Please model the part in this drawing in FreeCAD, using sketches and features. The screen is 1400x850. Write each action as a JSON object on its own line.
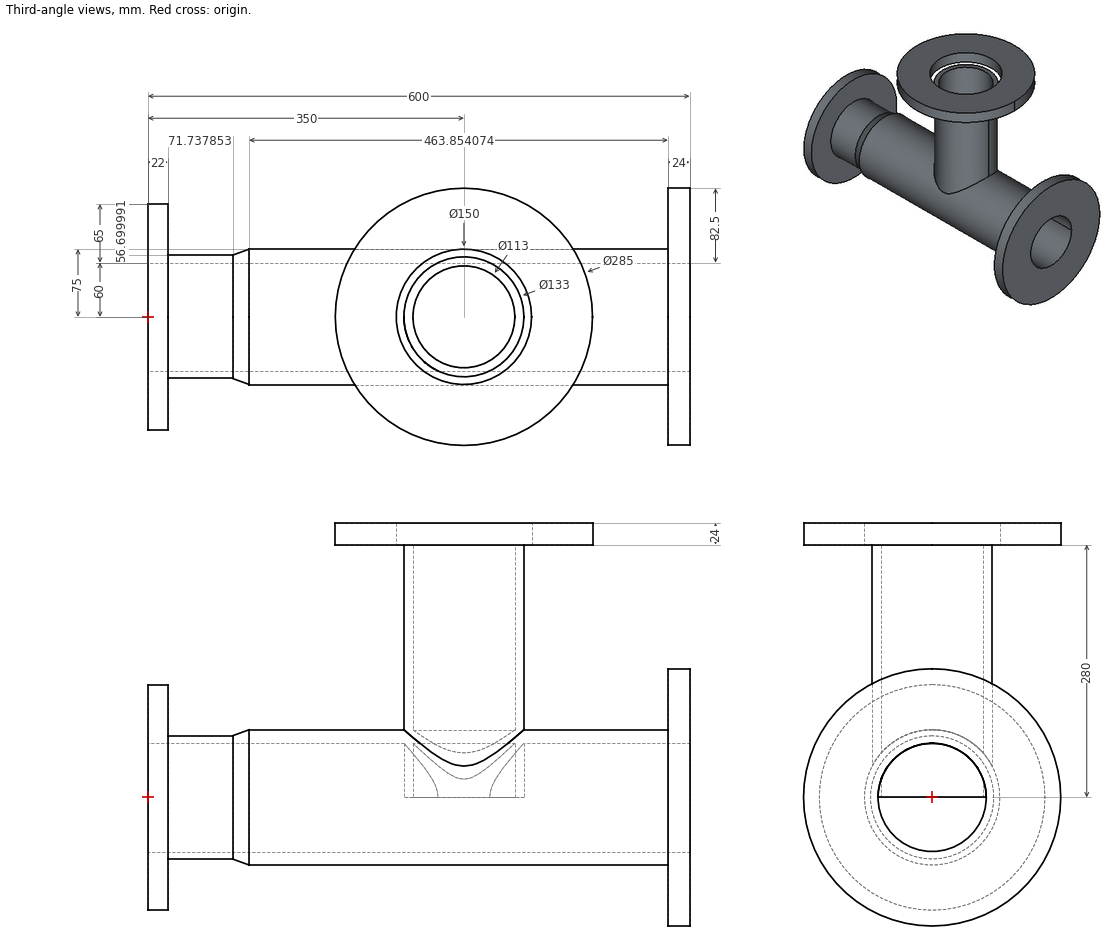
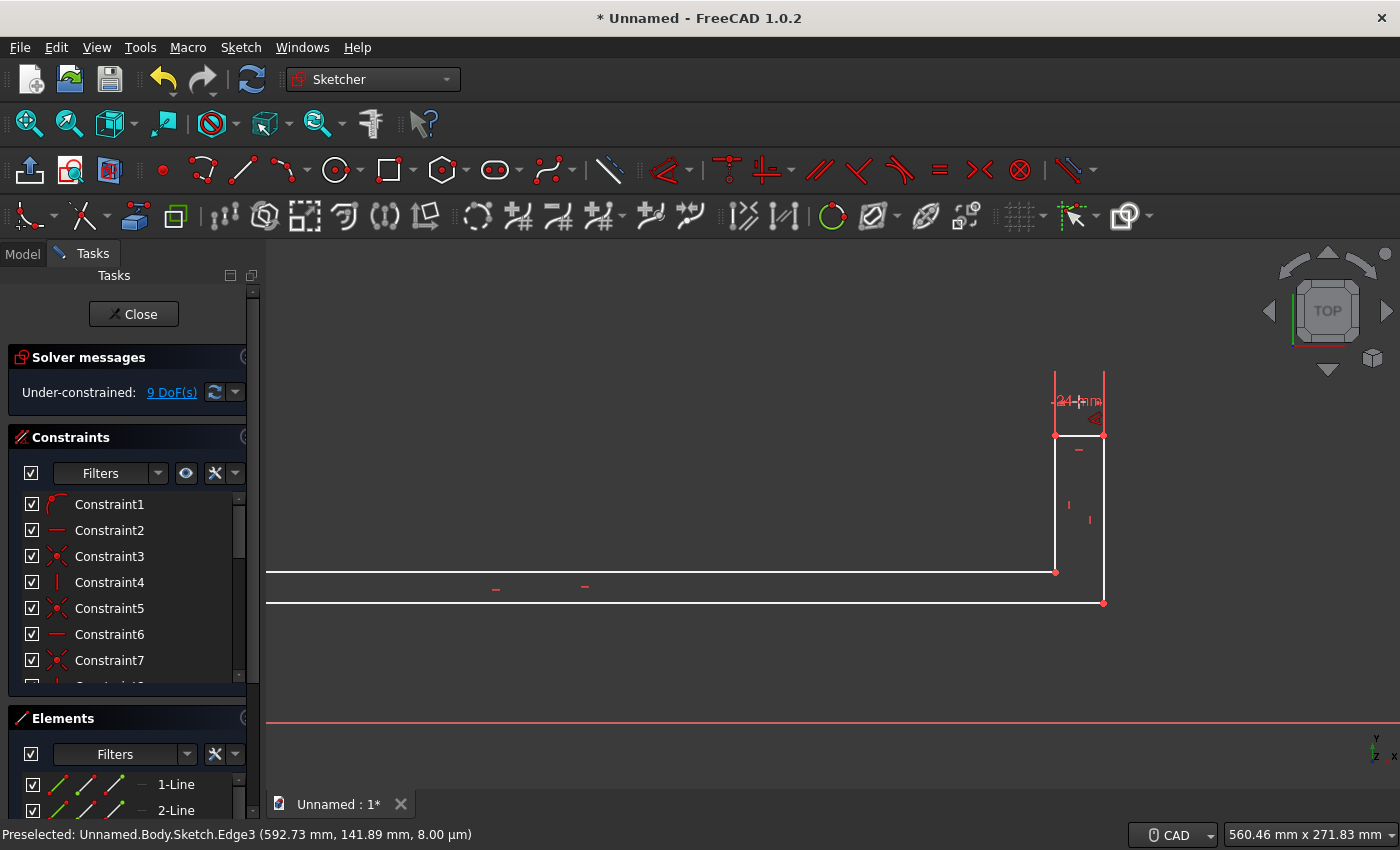
{"action": "scroll", "coordinate": [1090, 435], "scroll_direction": "down", "scroll_amount": 3}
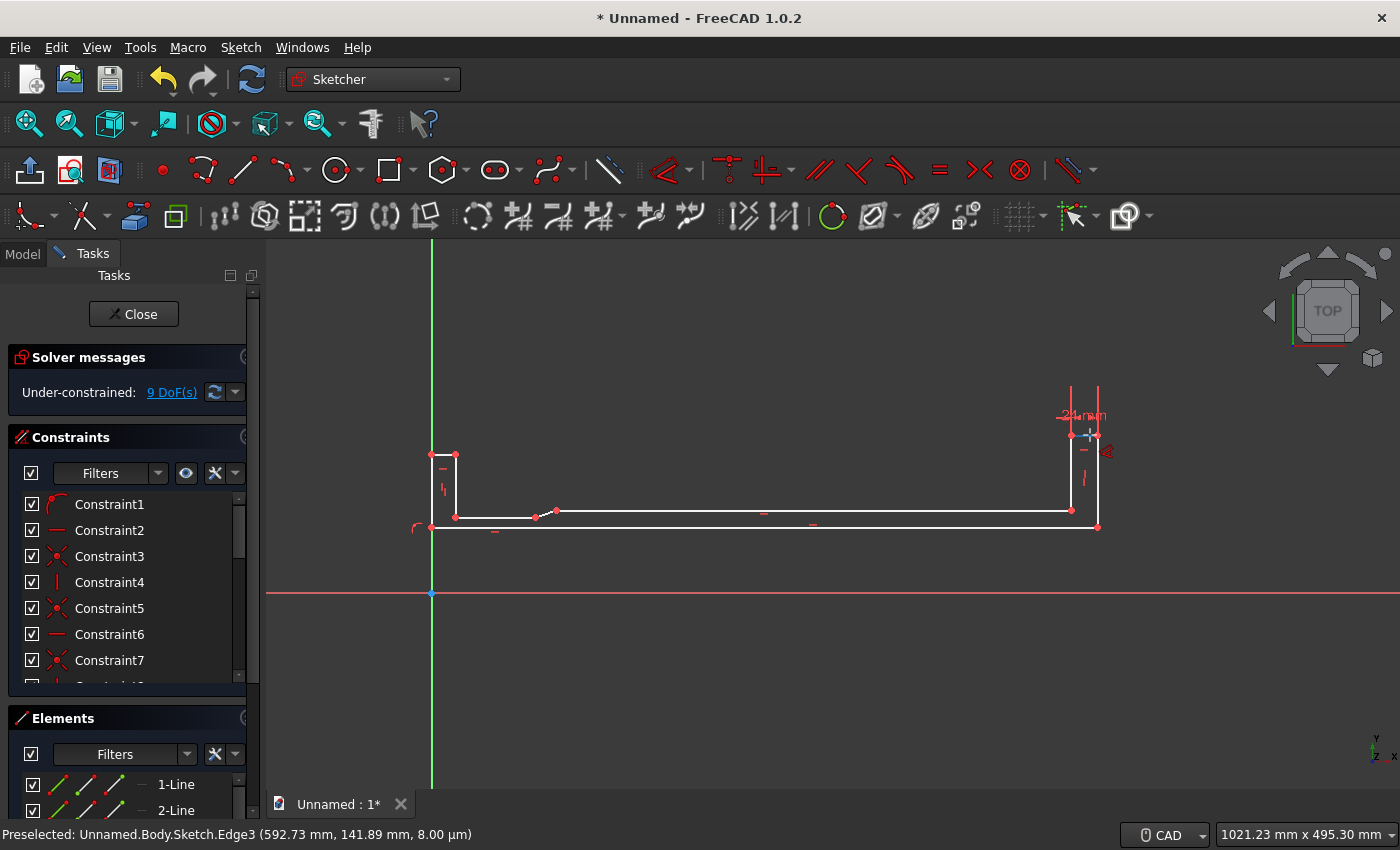
{"action": "scroll", "coordinate": [449, 455], "scroll_direction": "up", "scroll_amount": 4}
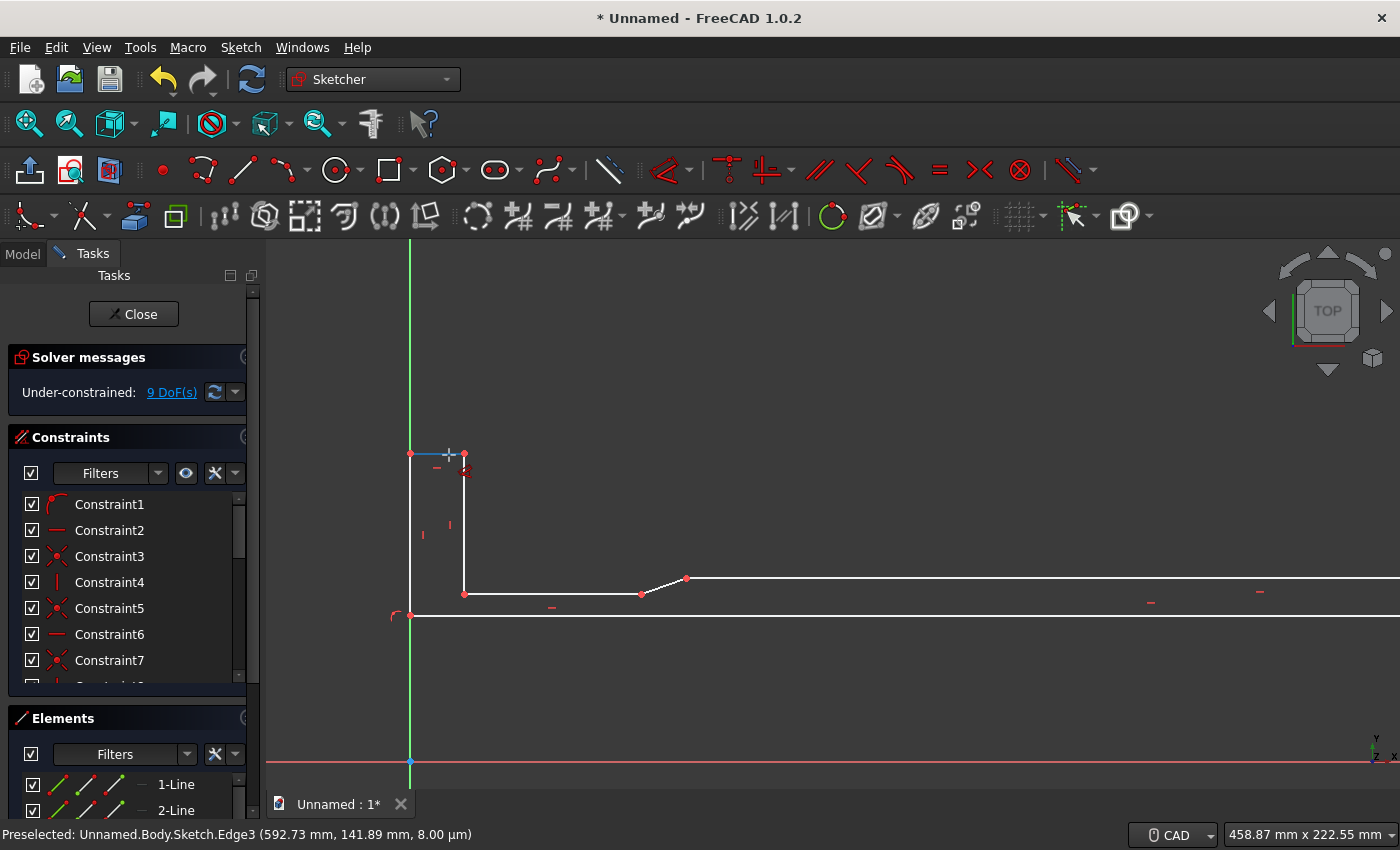
{"action": "left_click", "coordinate": [448, 454]}
{"action": "left_click", "coordinate": [437, 420]}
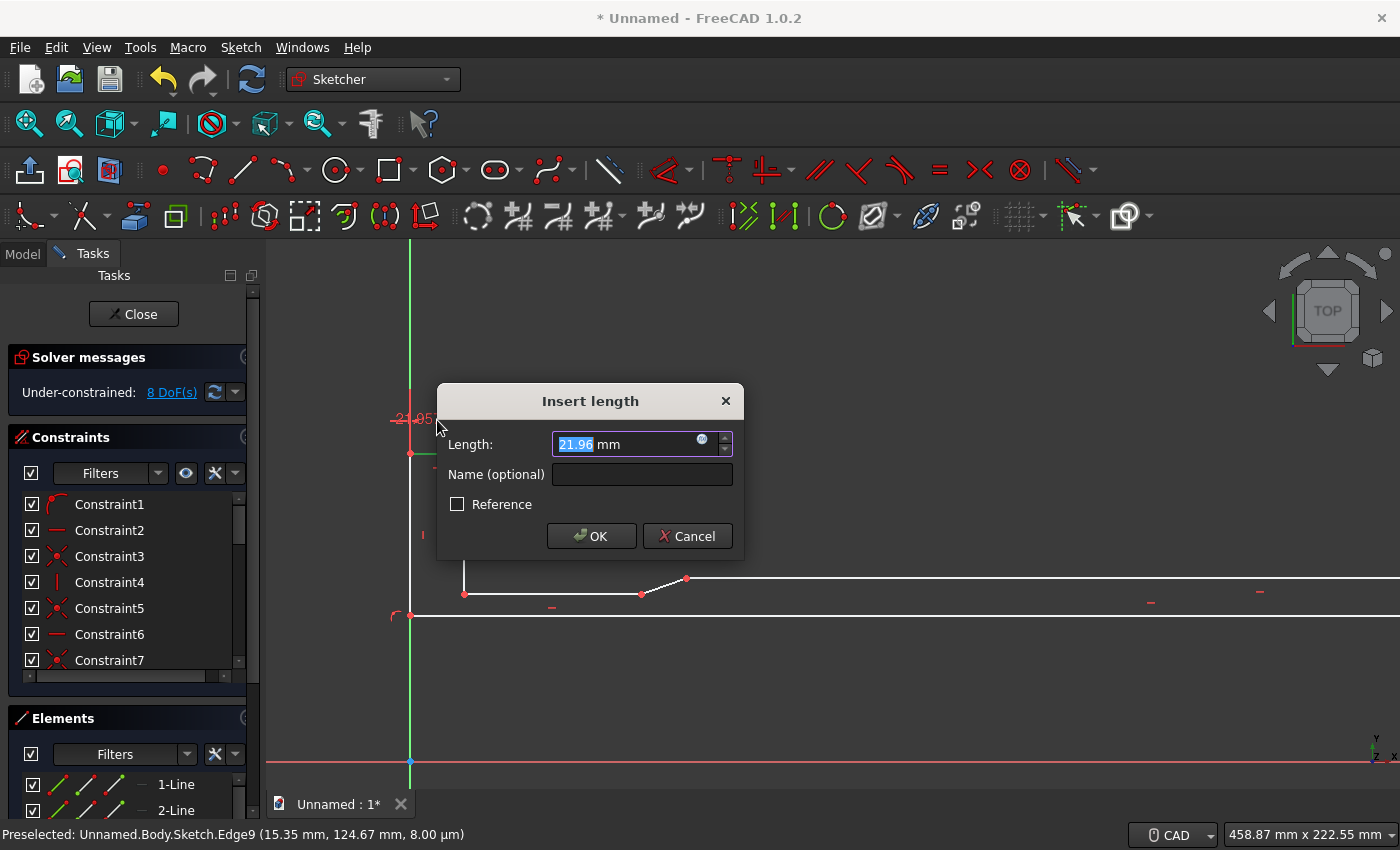
{"action": "type", "text": "22"}
{"action": "key", "text": "Return"}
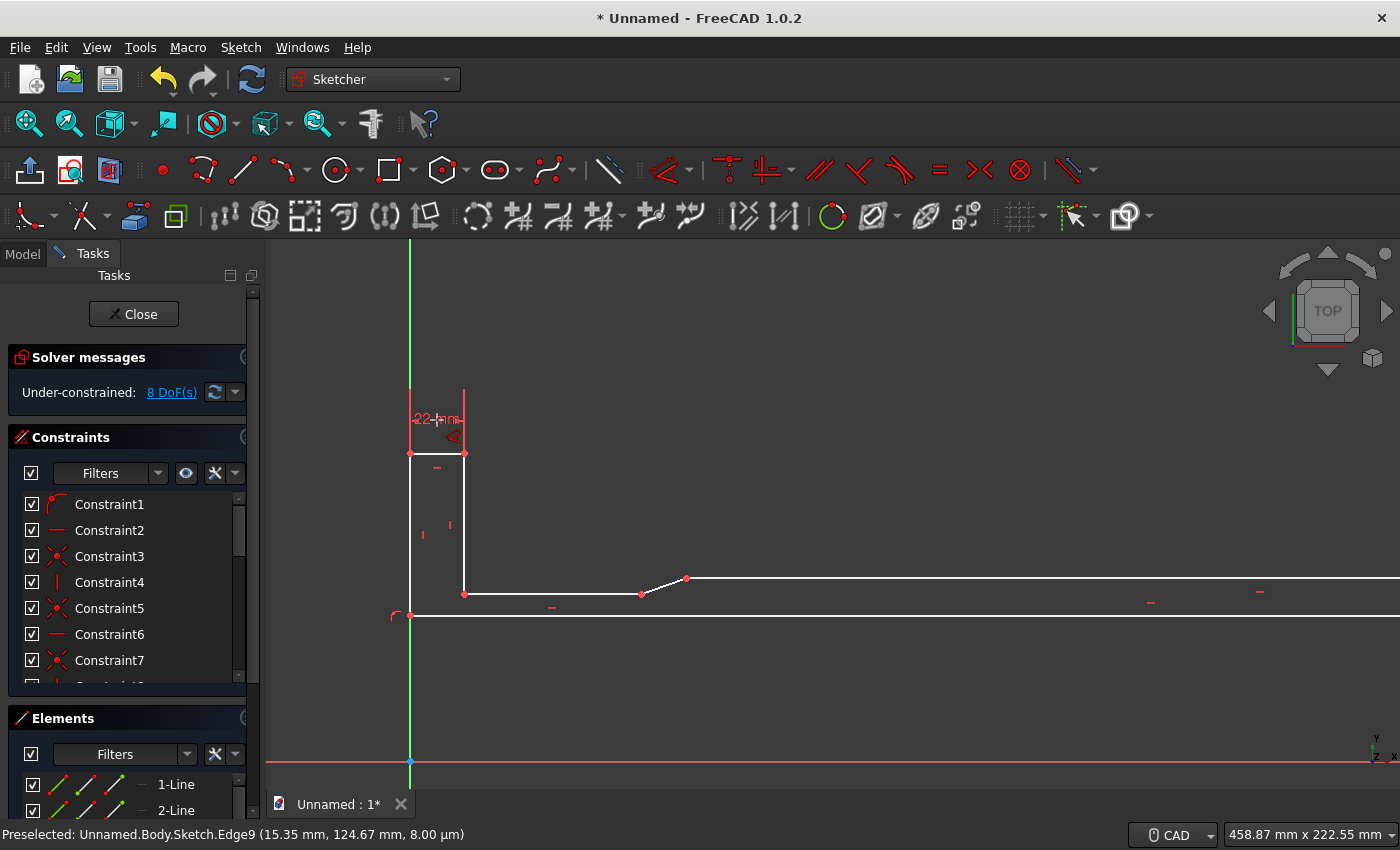
{"action": "left_click", "coordinate": [410, 502]}
{"action": "left_click", "coordinate": [376, 535]}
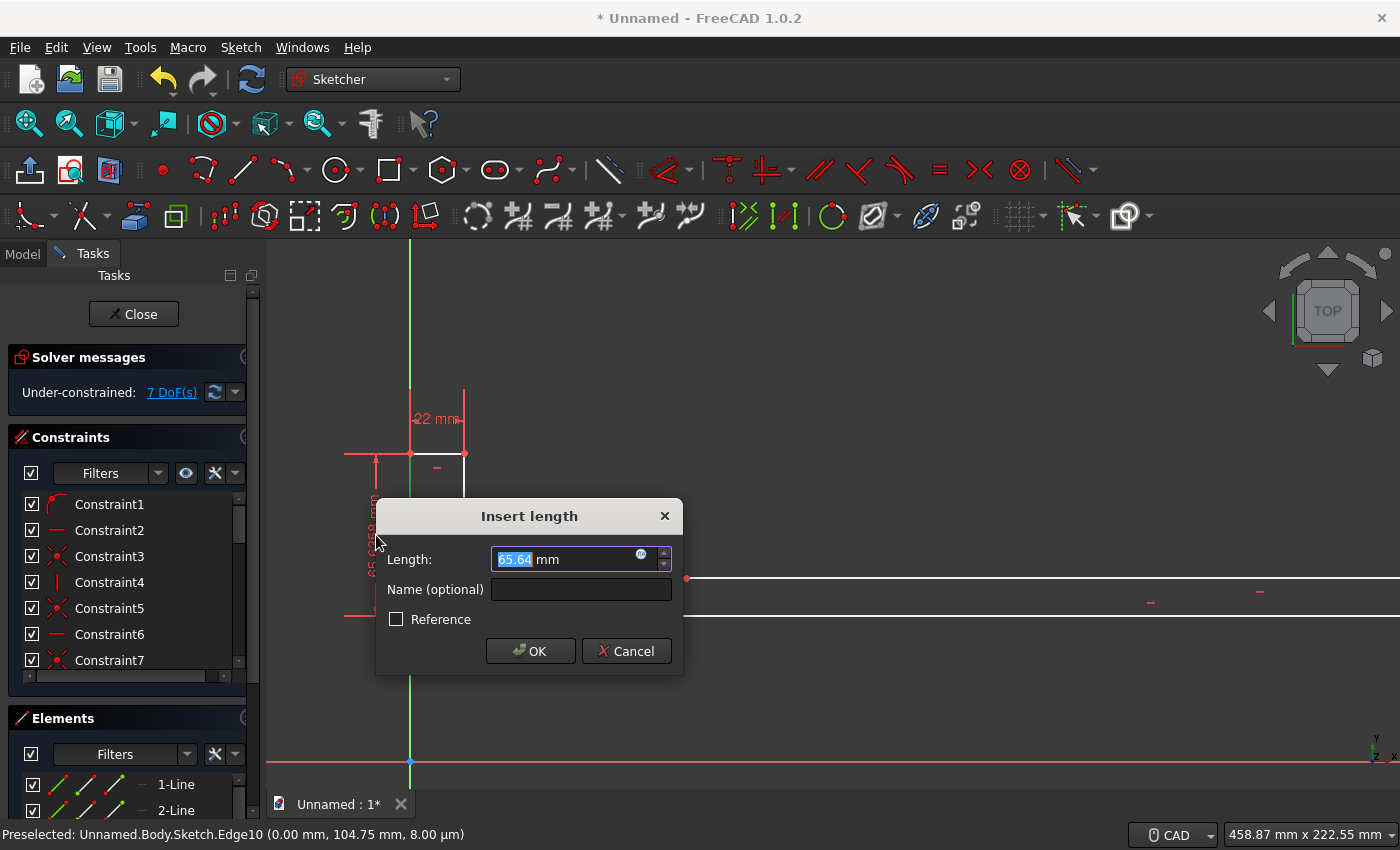
{"action": "type", "text": "65"}
{"action": "key", "text": "Return"}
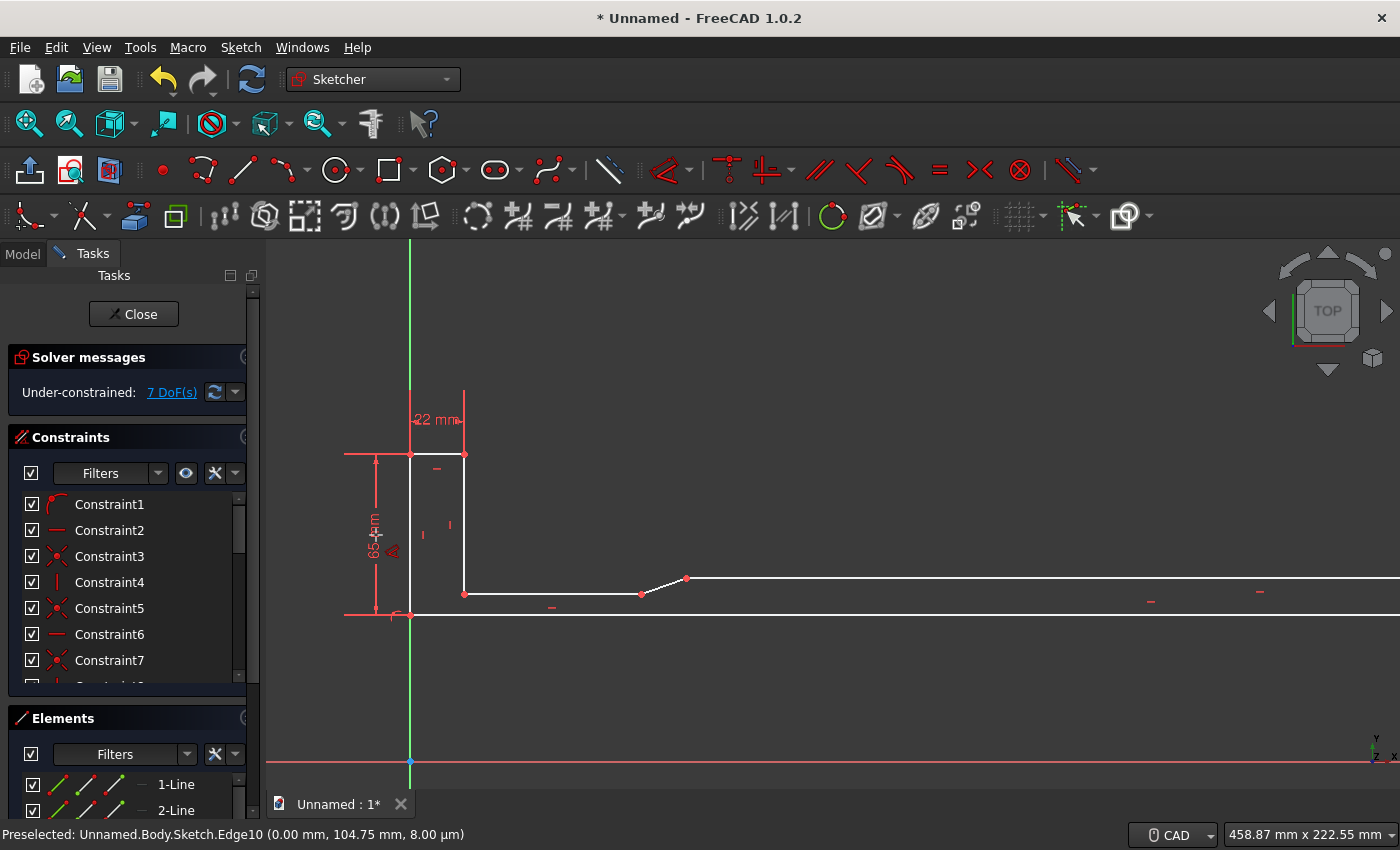
{"action": "left_click", "coordinate": [855, 615]}
{"action": "left_click", "coordinate": [823, 649]}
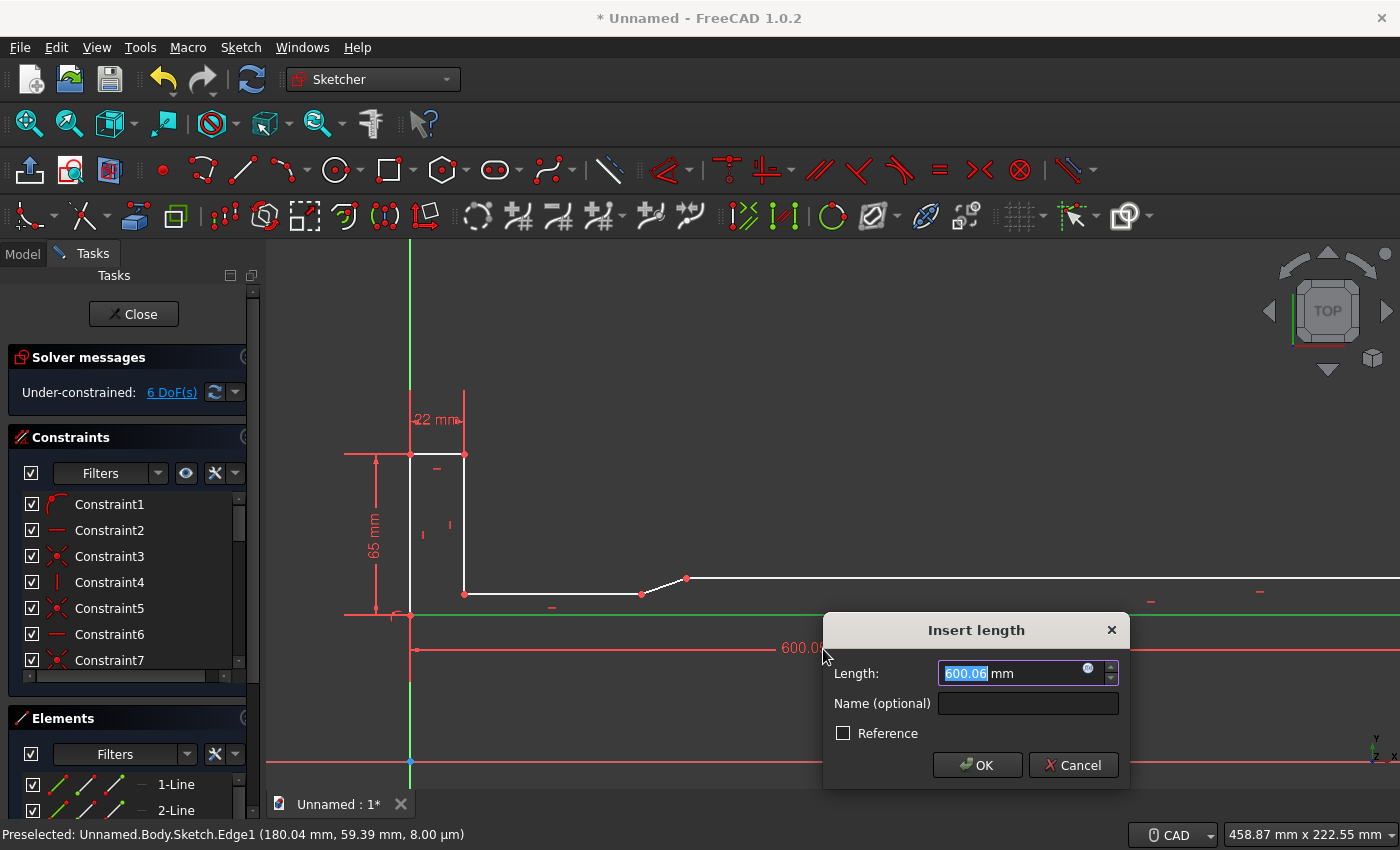
{"action": "type", "text": "600"}
{"action": "key", "text": "Return"}